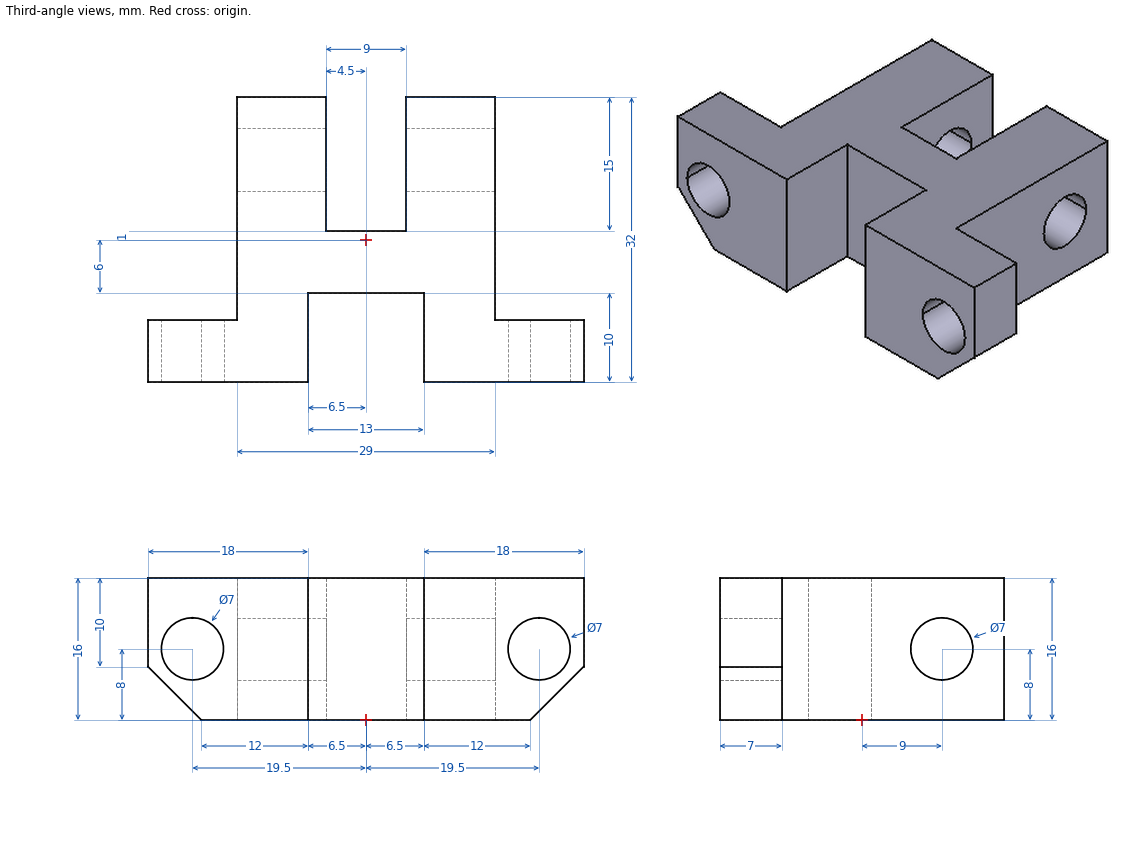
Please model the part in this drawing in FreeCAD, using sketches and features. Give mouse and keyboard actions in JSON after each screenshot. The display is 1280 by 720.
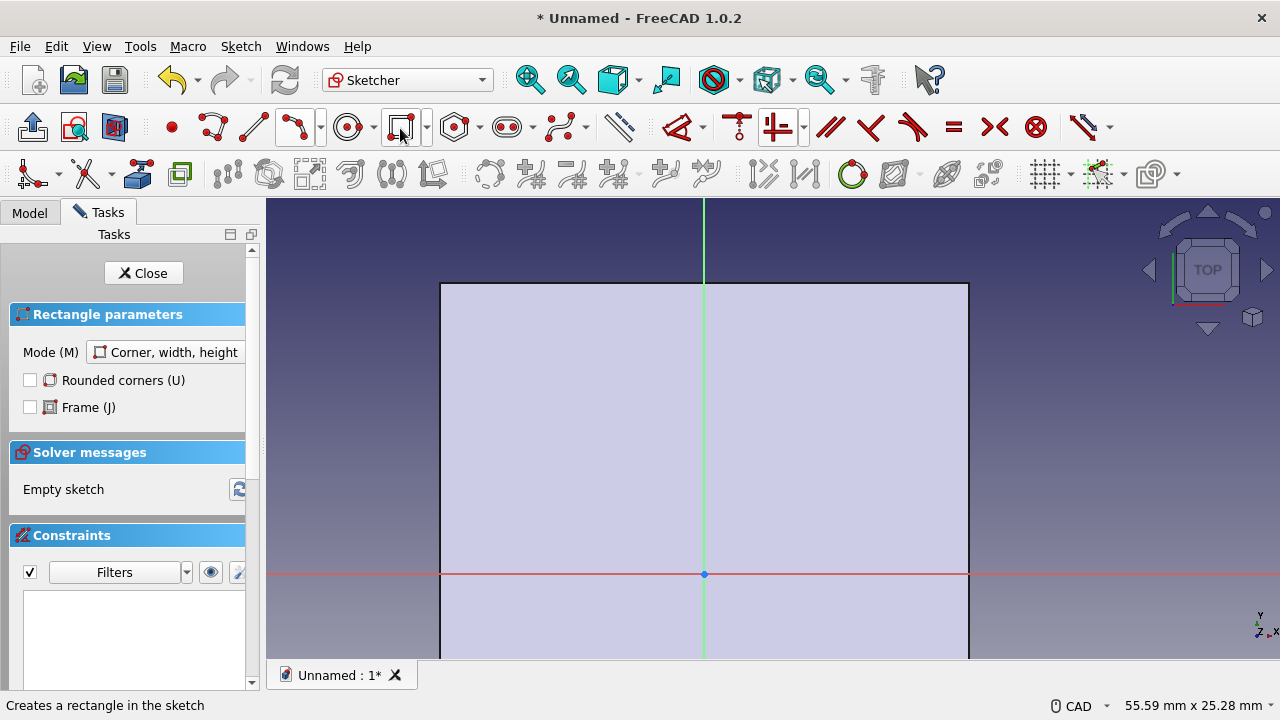
{"action": "left_click", "coordinate": [622, 283]}
{"action": "mouse_move", "coordinate": [786, 556]}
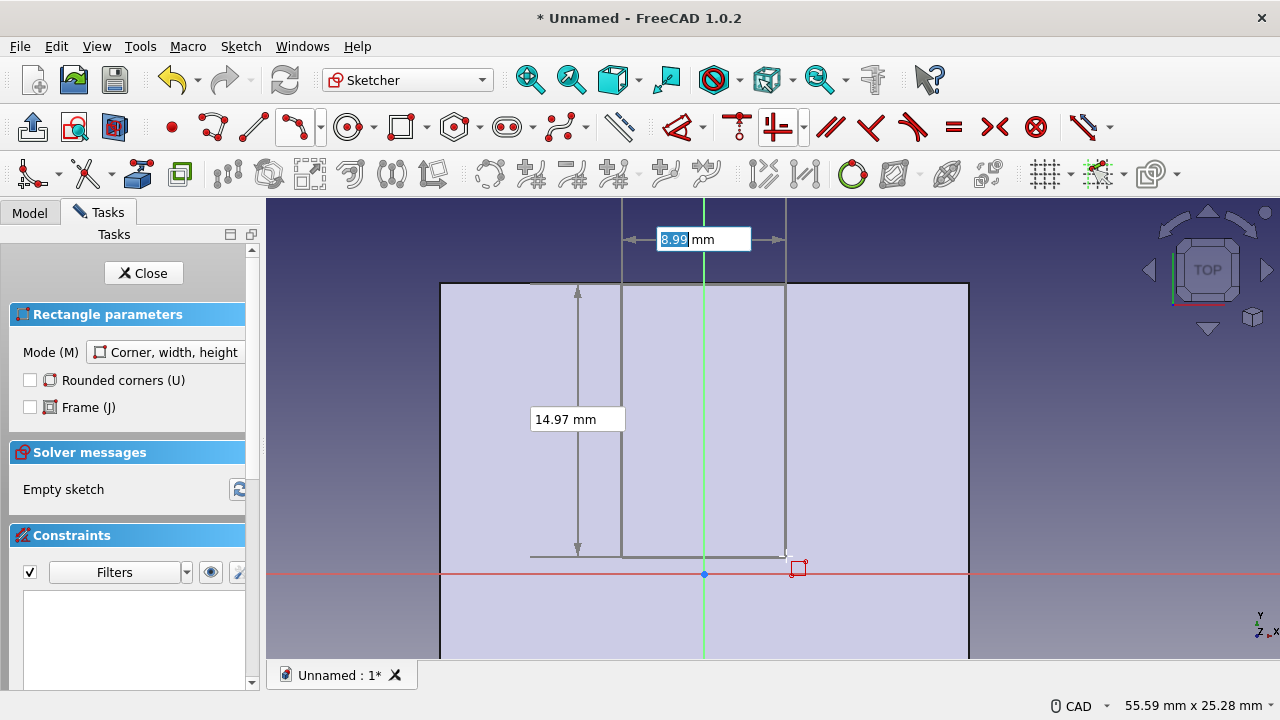
{"action": "type", "text": "9"}
{"action": "key", "text": "Tab"}
{"action": "type", "text": "15"}
{"action": "key", "text": "Return"}
{"action": "key", "text": "Escape"}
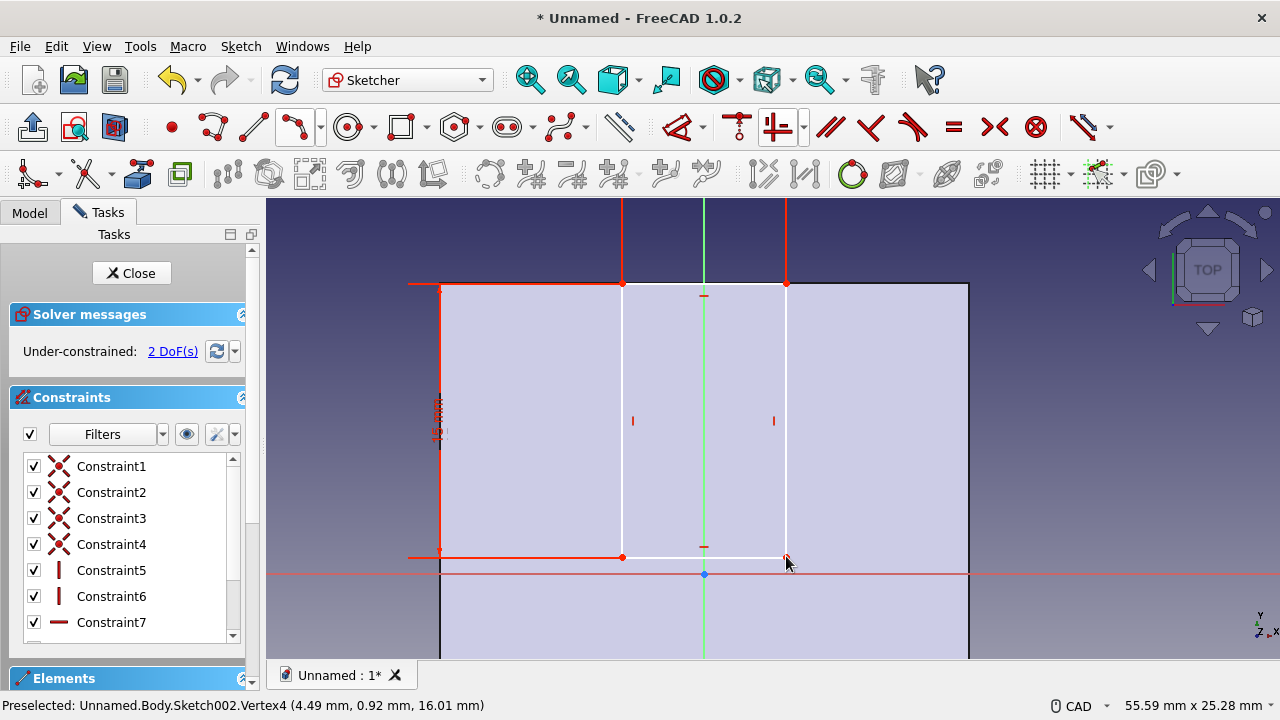
{"action": "left_click", "coordinate": [676, 128]}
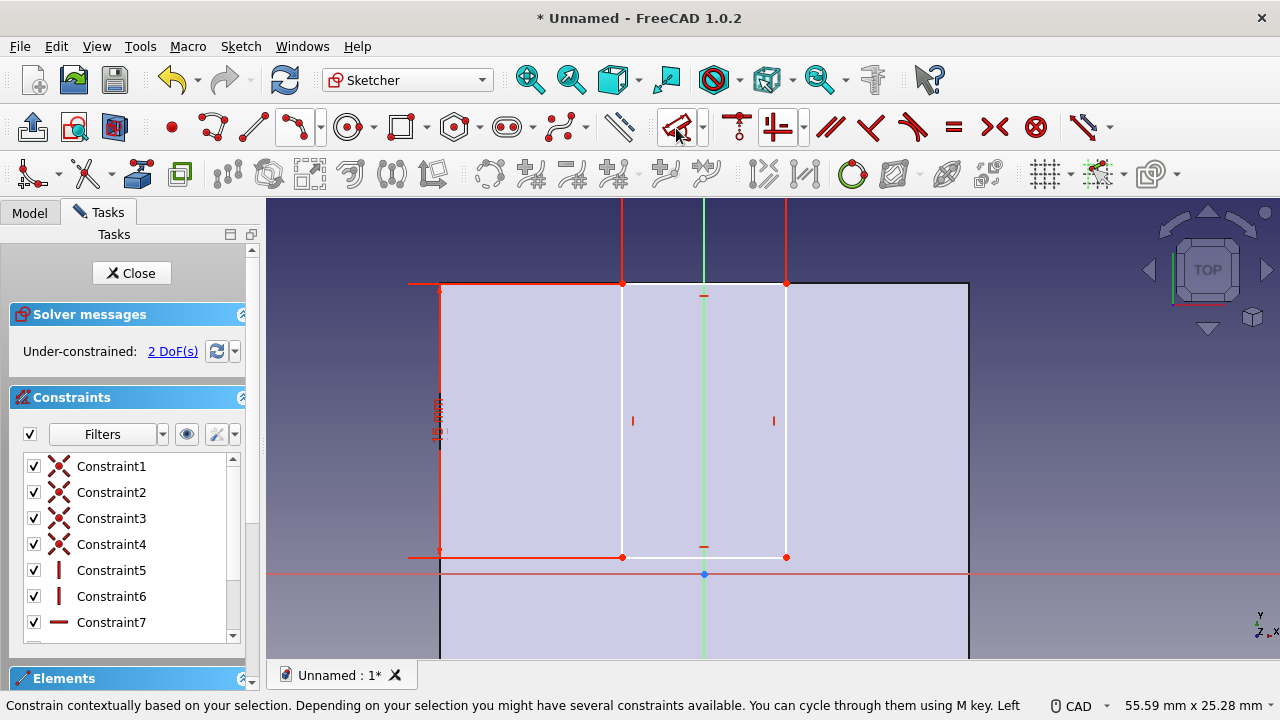
{"action": "scroll", "coordinate": [622, 558], "scroll_direction": "up", "scroll_amount": 4}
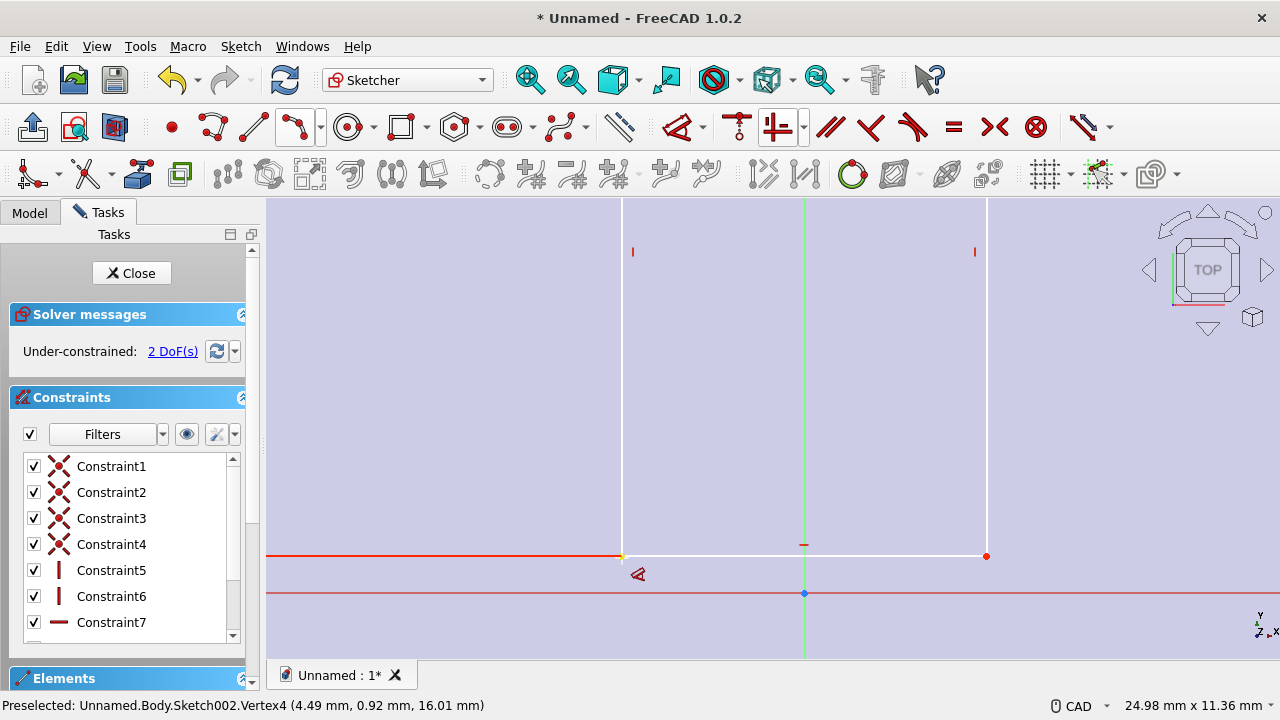
{"action": "left_click", "coordinate": [622, 556]}
{"action": "left_click", "coordinate": [588, 575]}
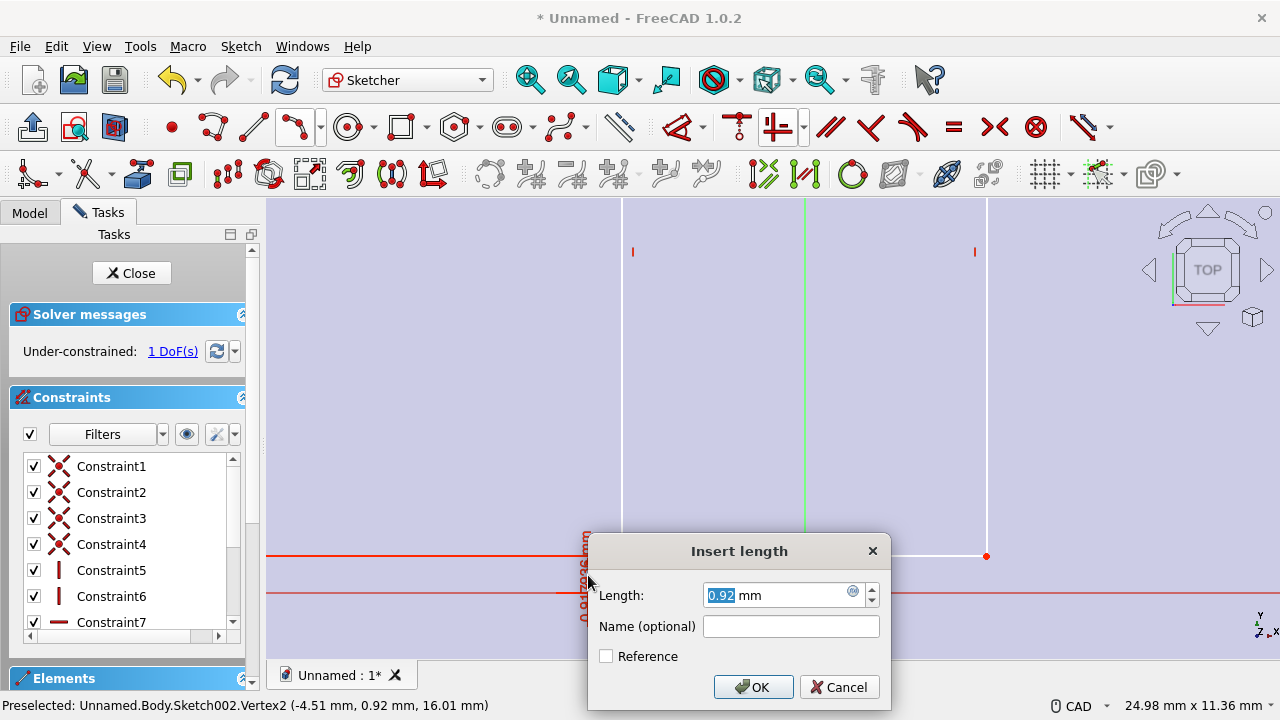
{"action": "type", "text": "1"}
{"action": "key", "text": "Return"}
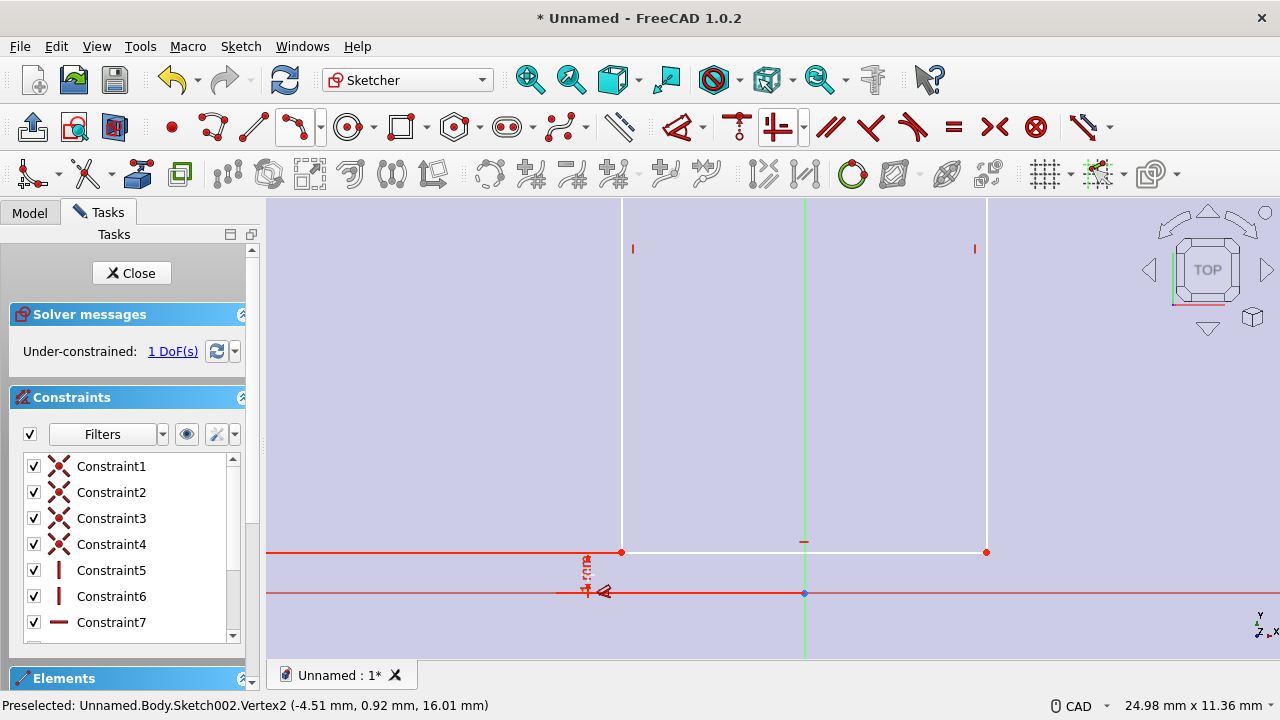
{"action": "scroll", "coordinate": [623, 559], "scroll_direction": "down", "scroll_amount": 4}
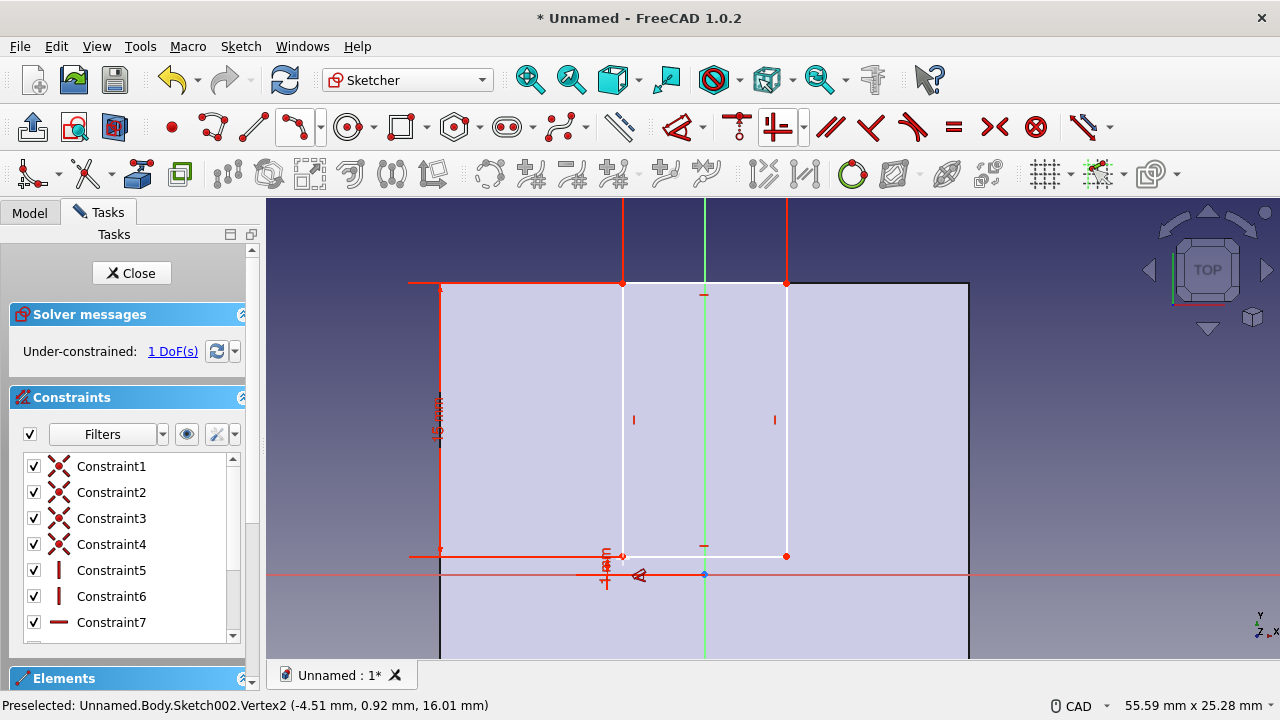
{"action": "left_click", "coordinate": [623, 283]}
{"action": "left_click", "coordinate": [664, 609]}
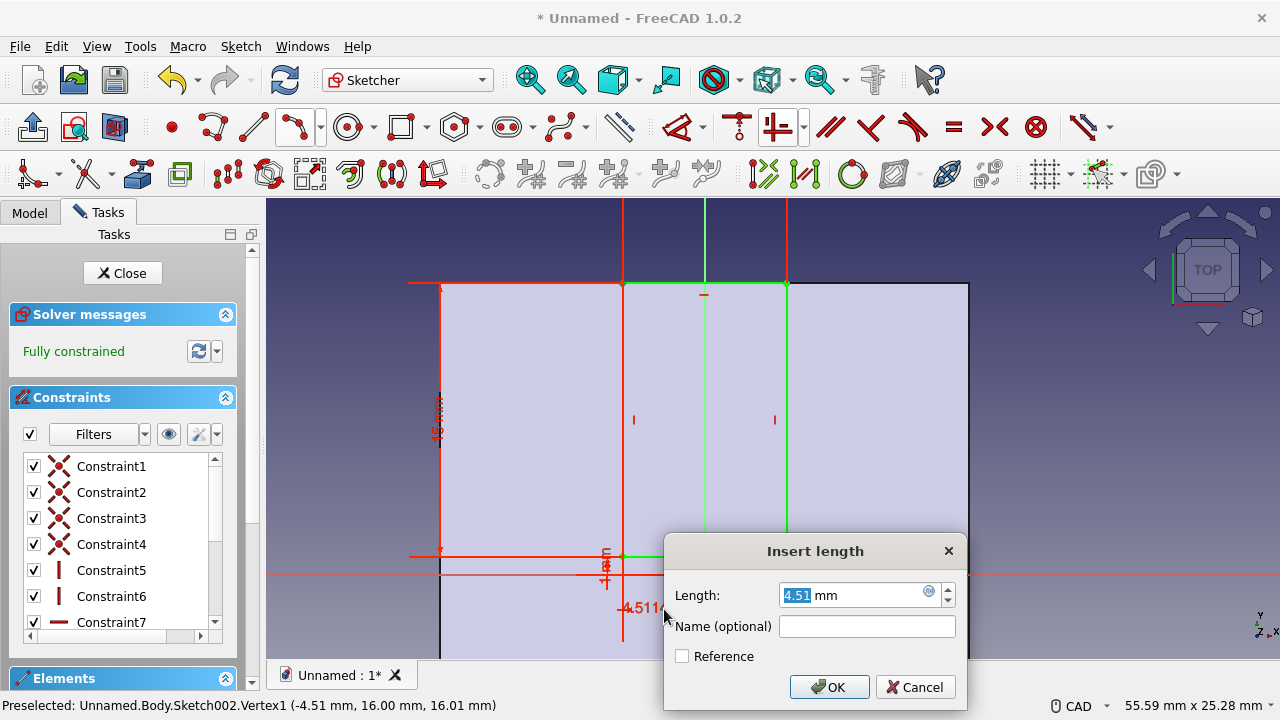
{"action": "type", "text": "4.5"}
{"action": "key", "text": "Return"}
{"action": "key", "text": "Escape"}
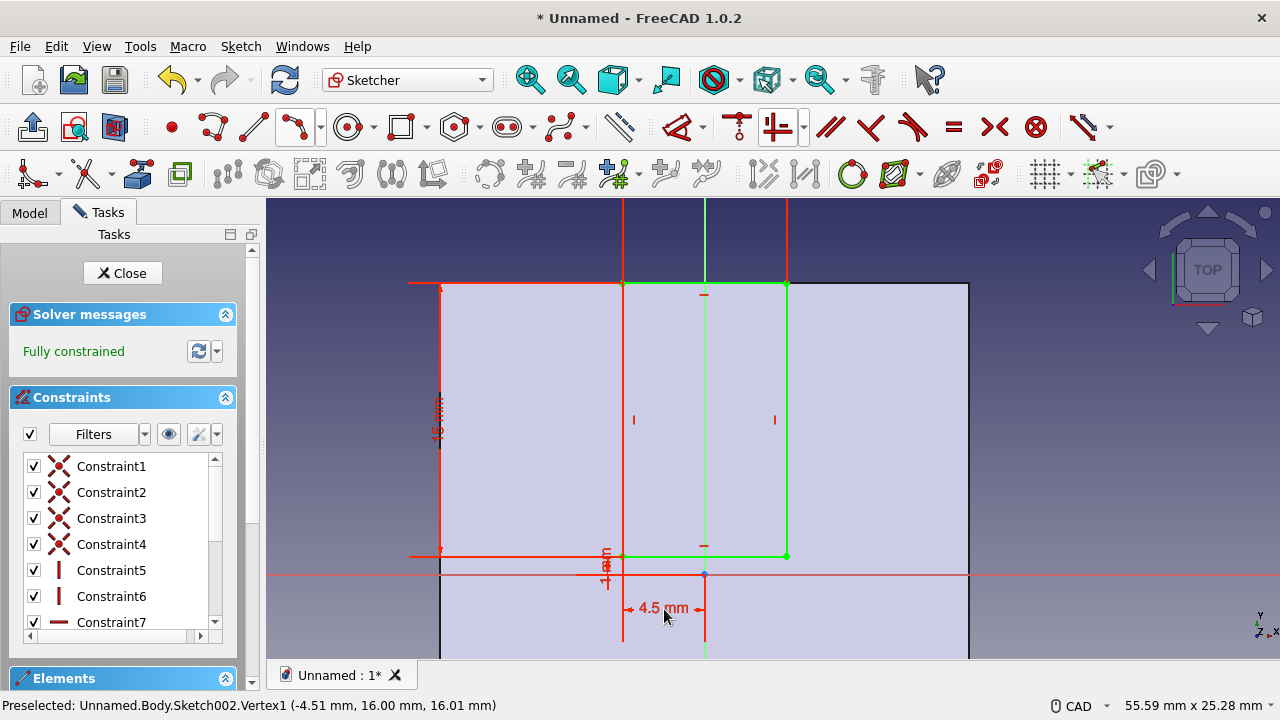
{"action": "left_click", "coordinate": [123, 273]}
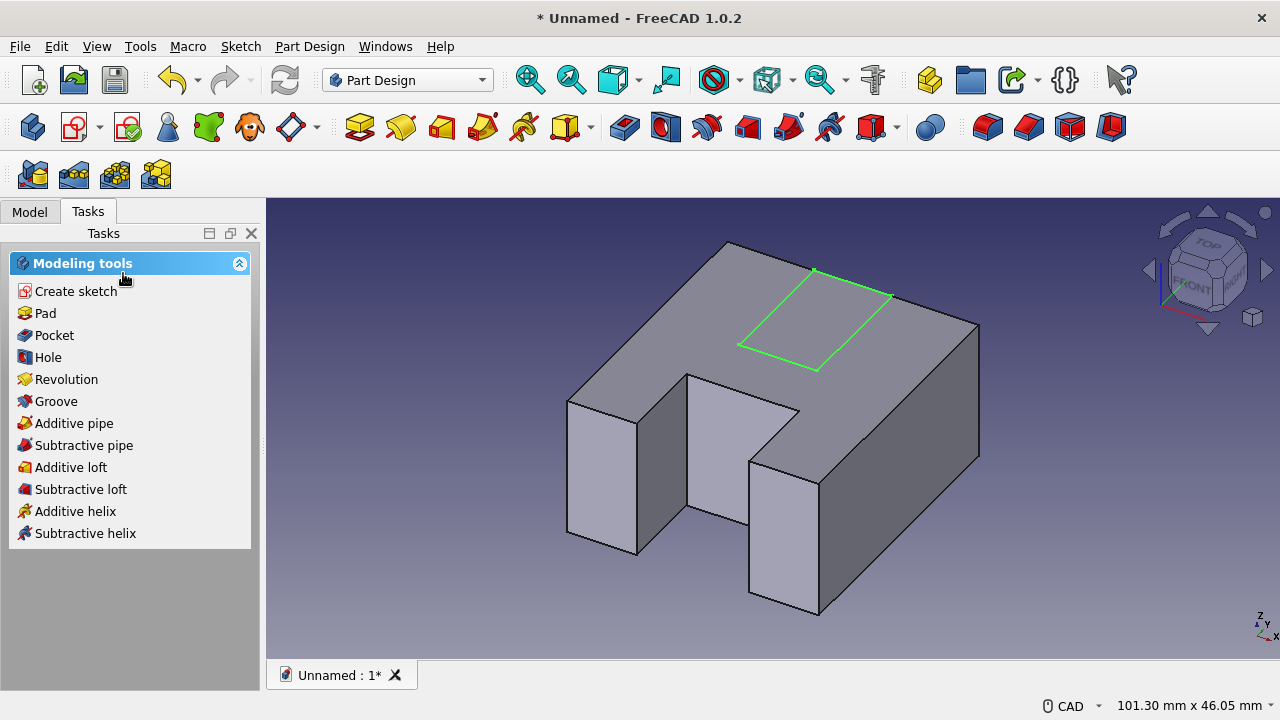
{"action": "left_click", "coordinate": [625, 128]}